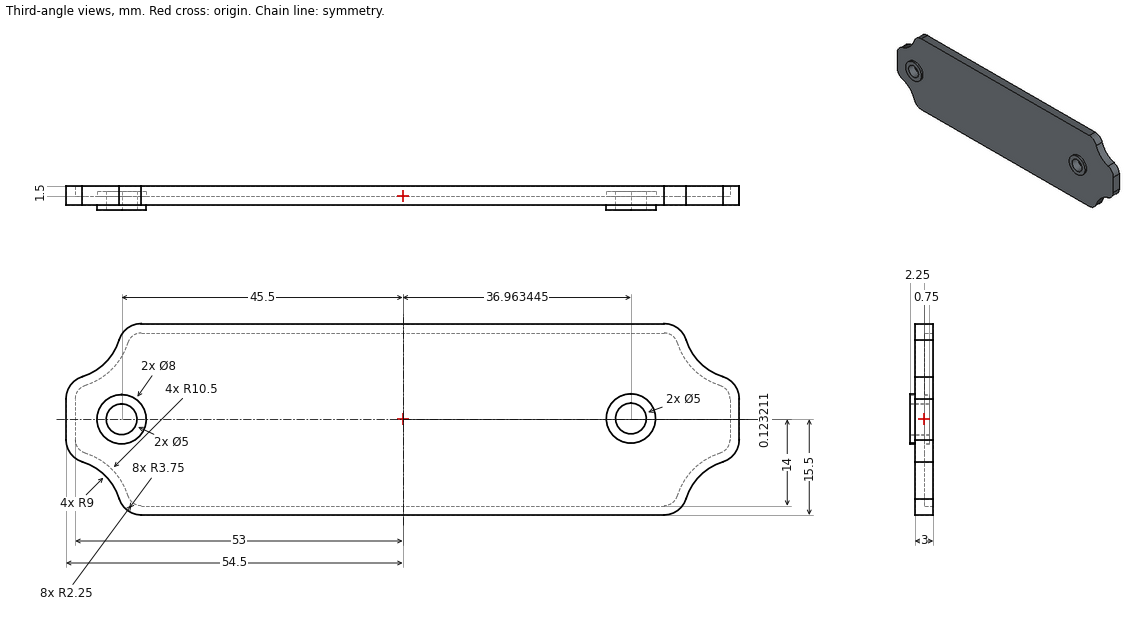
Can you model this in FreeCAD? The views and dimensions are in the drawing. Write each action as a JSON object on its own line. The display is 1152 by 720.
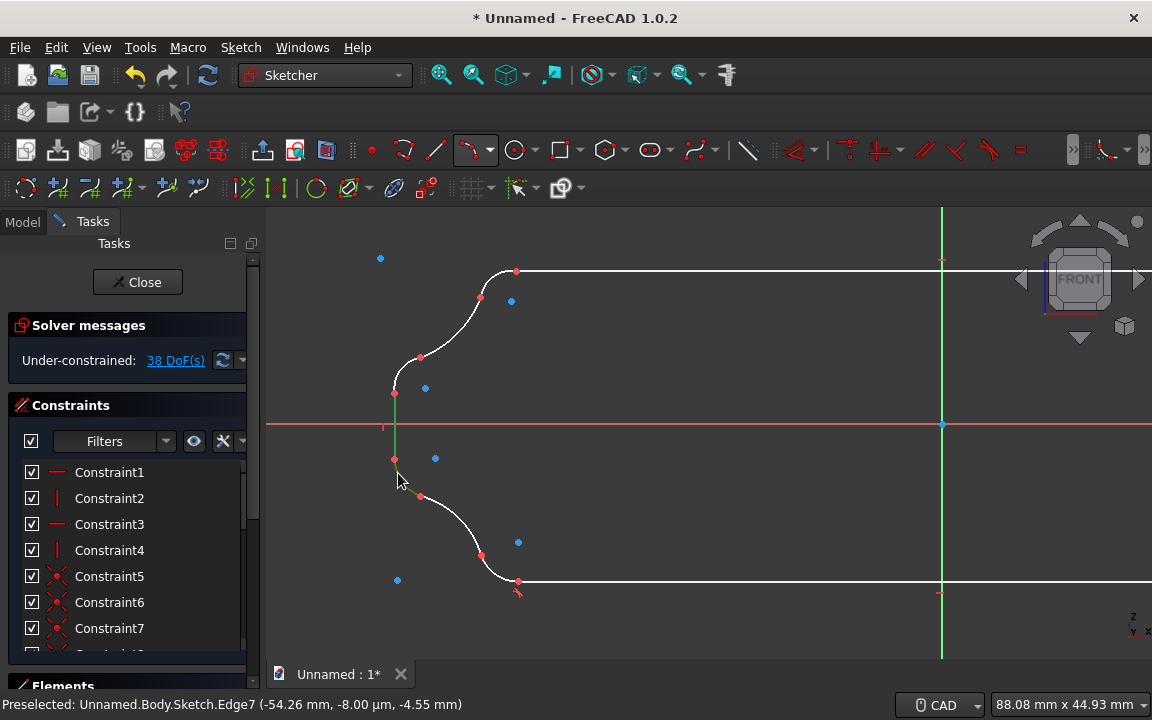
{"action": "left_click", "coordinate": [990, 150]}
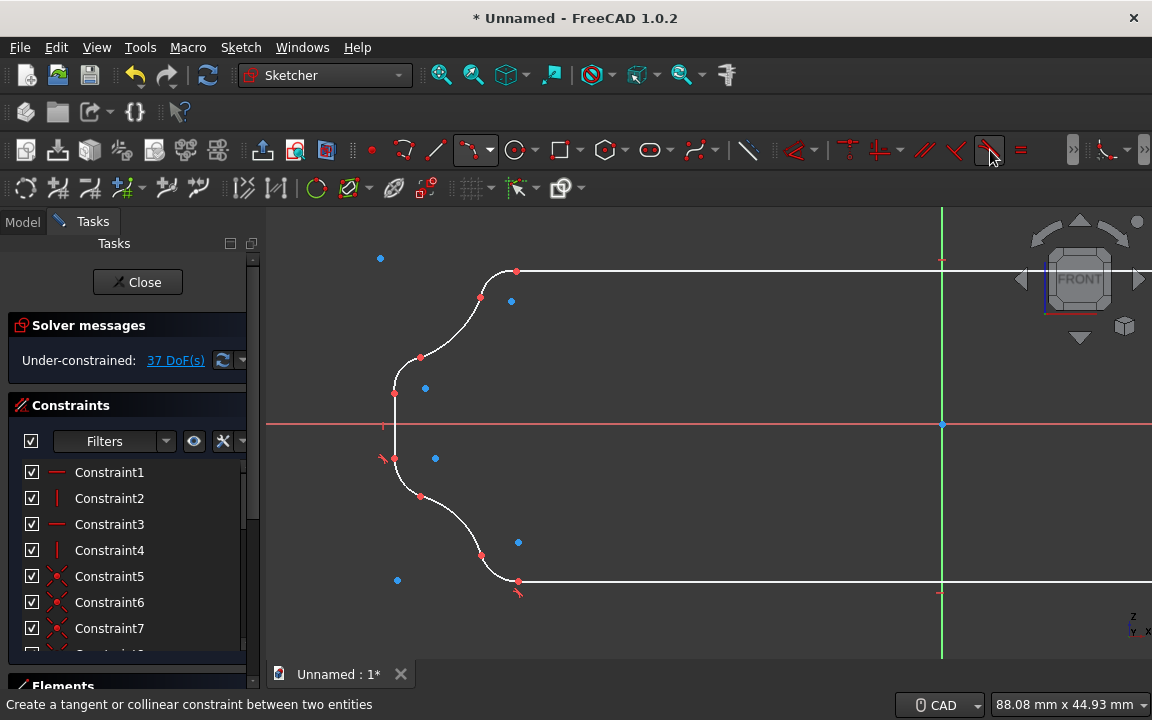
{"action": "left_click", "coordinate": [395, 439]}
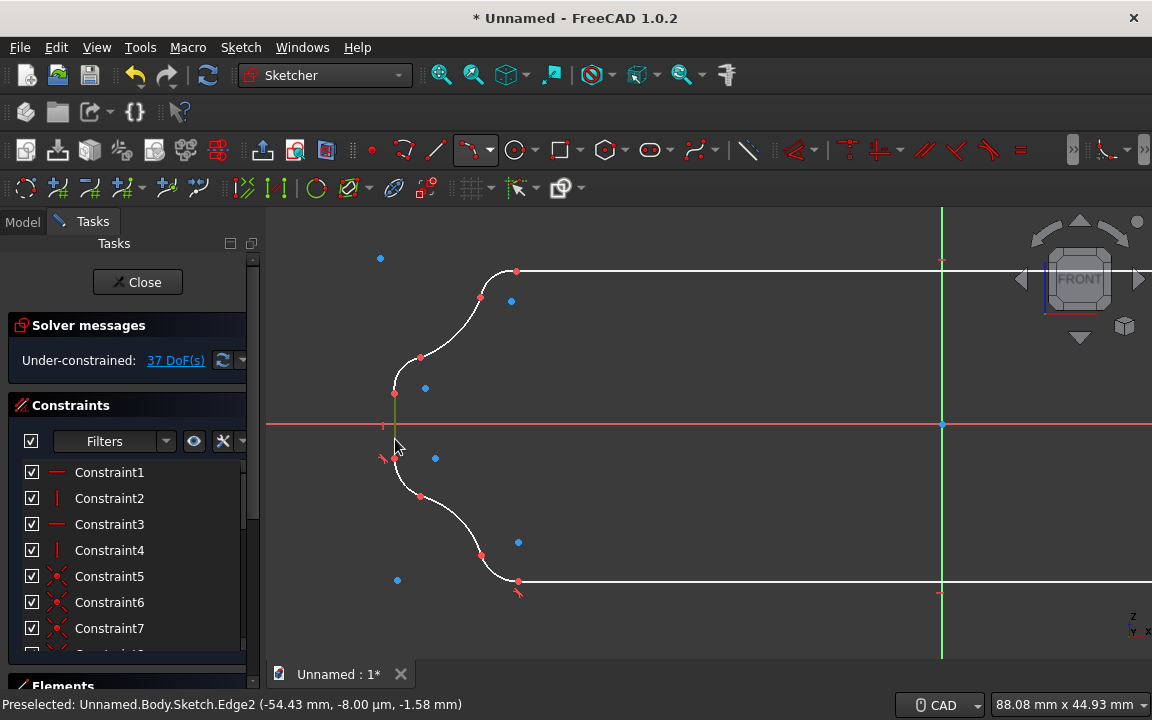
{"action": "left_click", "coordinate": [407, 363]}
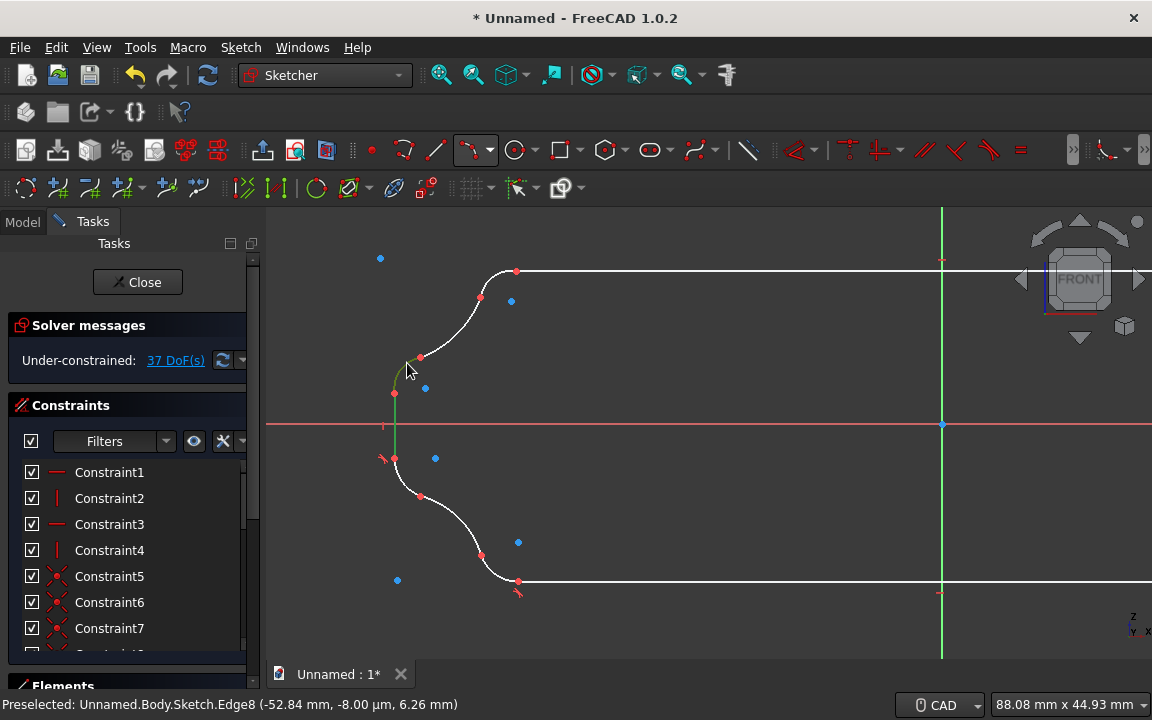
{"action": "left_click", "coordinate": [990, 150]}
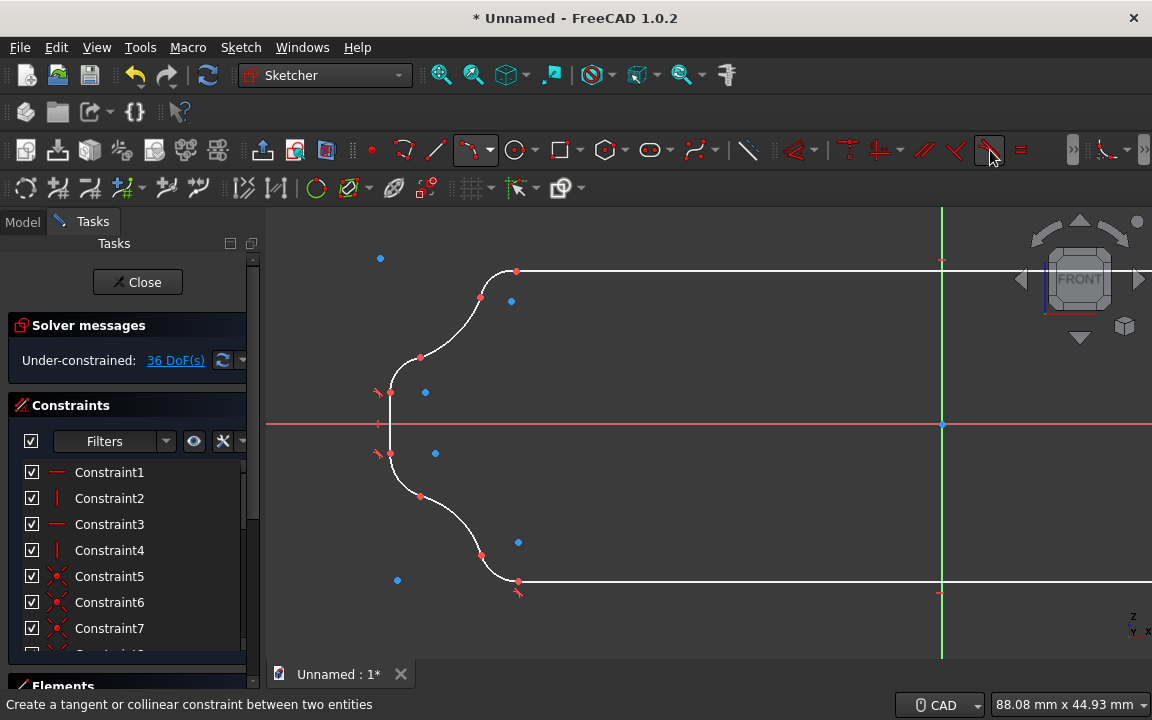
{"action": "left_click", "coordinate": [772, 271]}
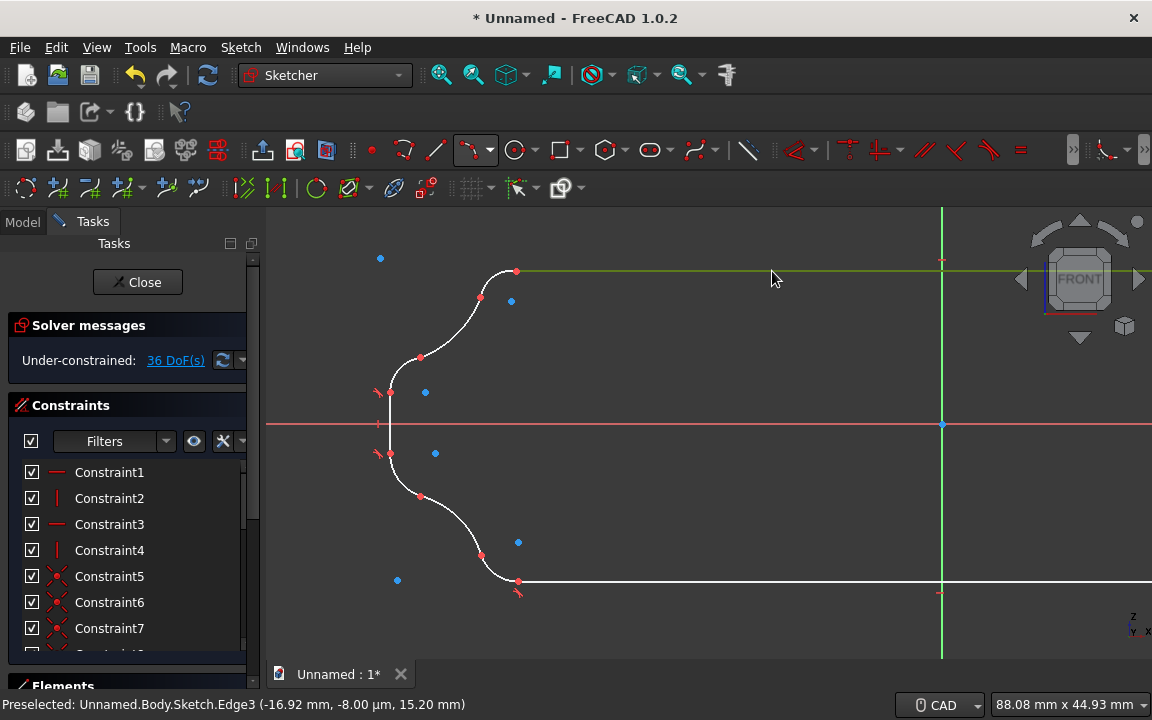
{"action": "left_click", "coordinate": [502, 272]}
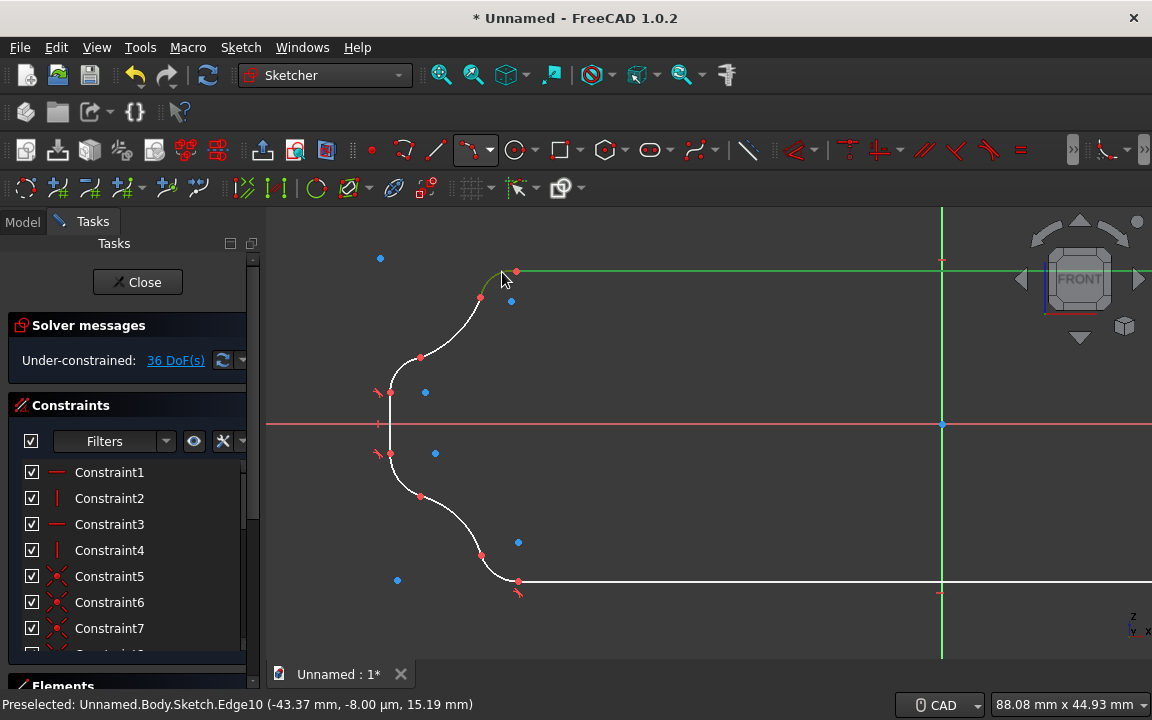
{"action": "left_click", "coordinate": [990, 150]}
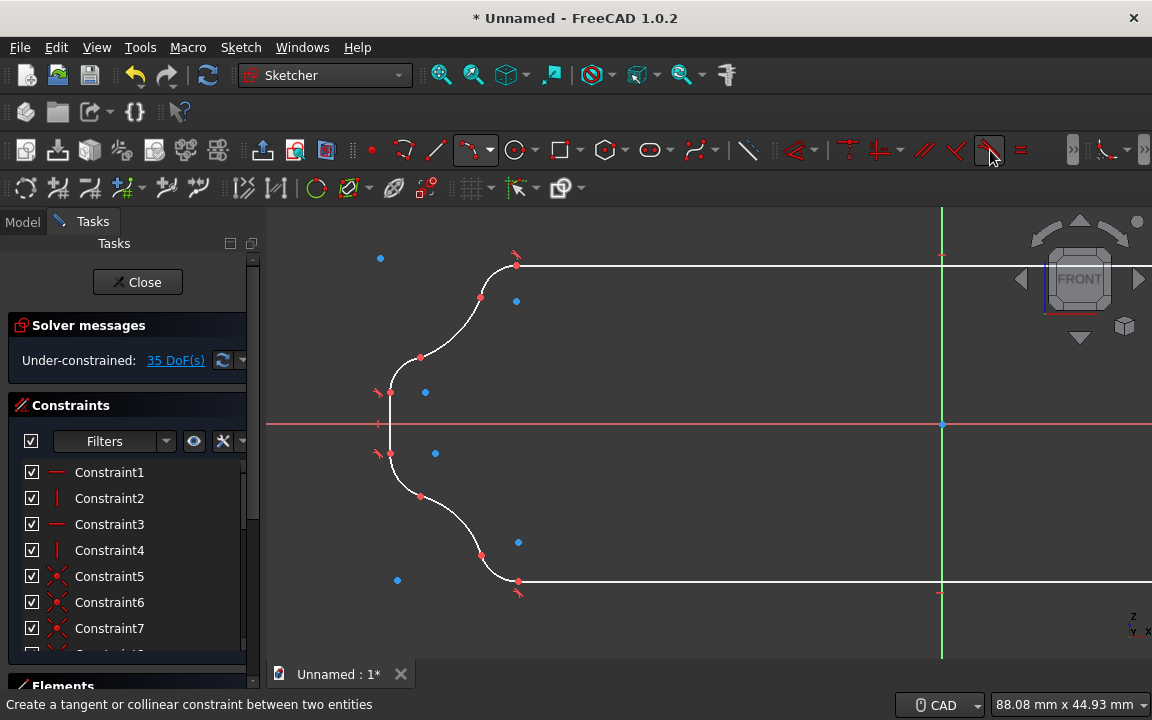
{"action": "left_click", "coordinate": [772, 266]}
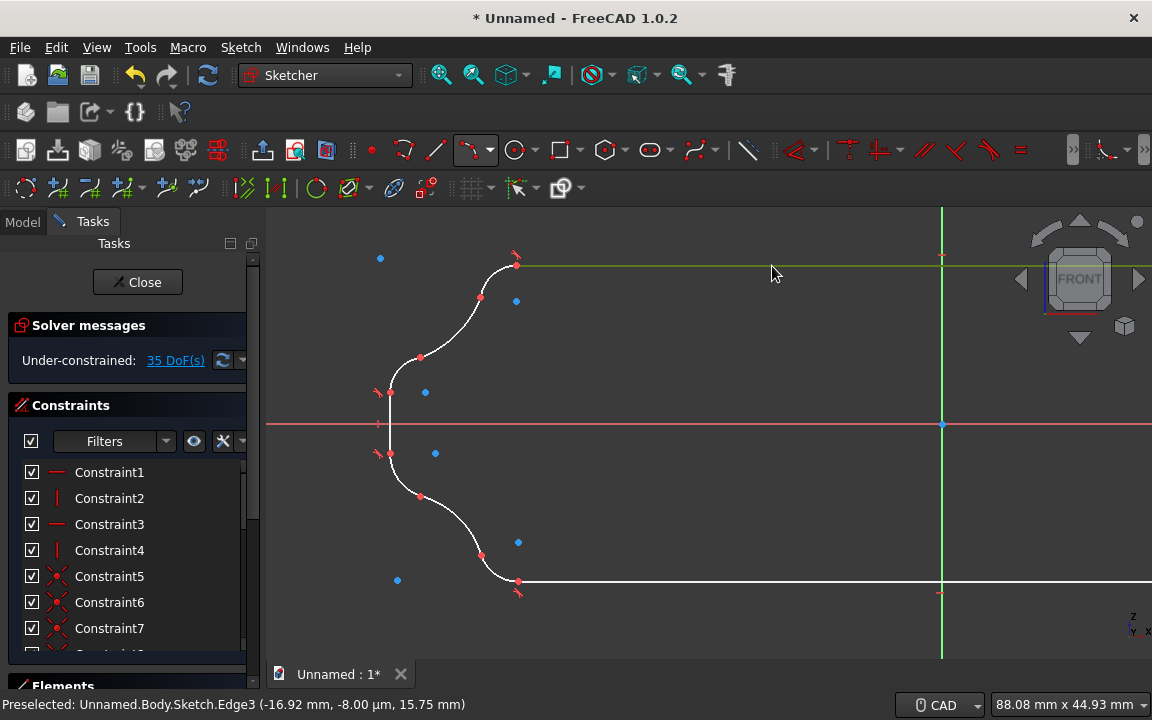
{"action": "scroll", "coordinate": [394, 440], "scroll_direction": "down", "scroll_amount": 4}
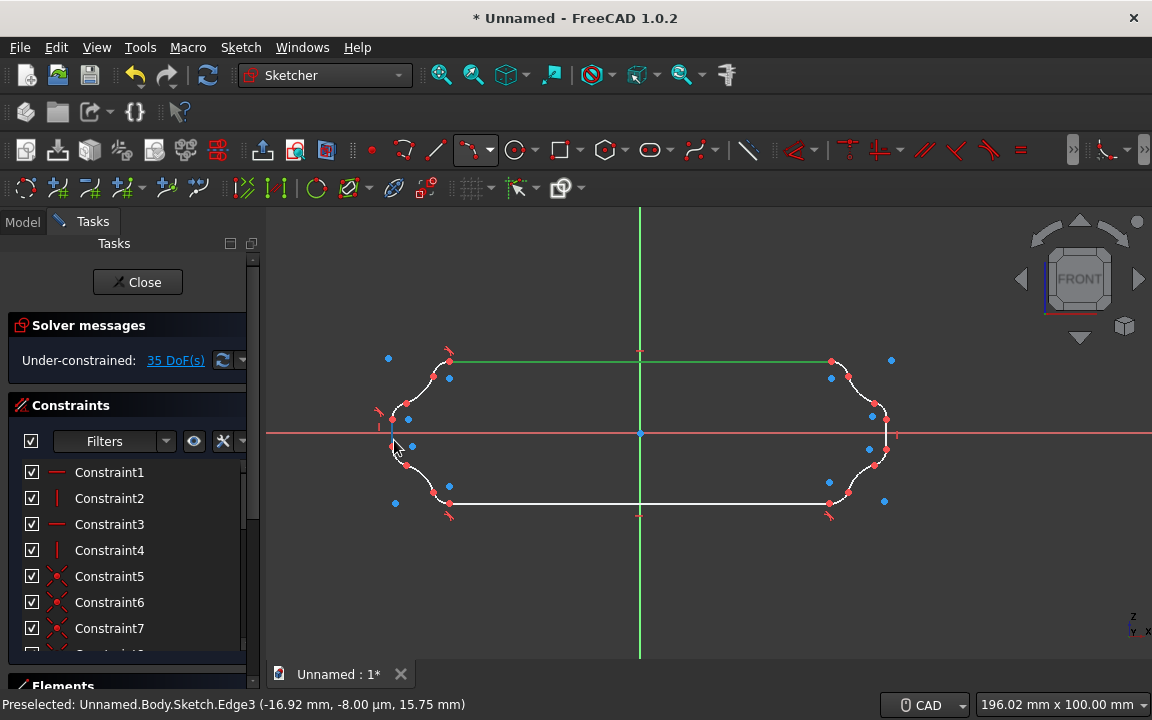
{"action": "scroll", "coordinate": [846, 370], "scroll_direction": "up", "scroll_amount": 4}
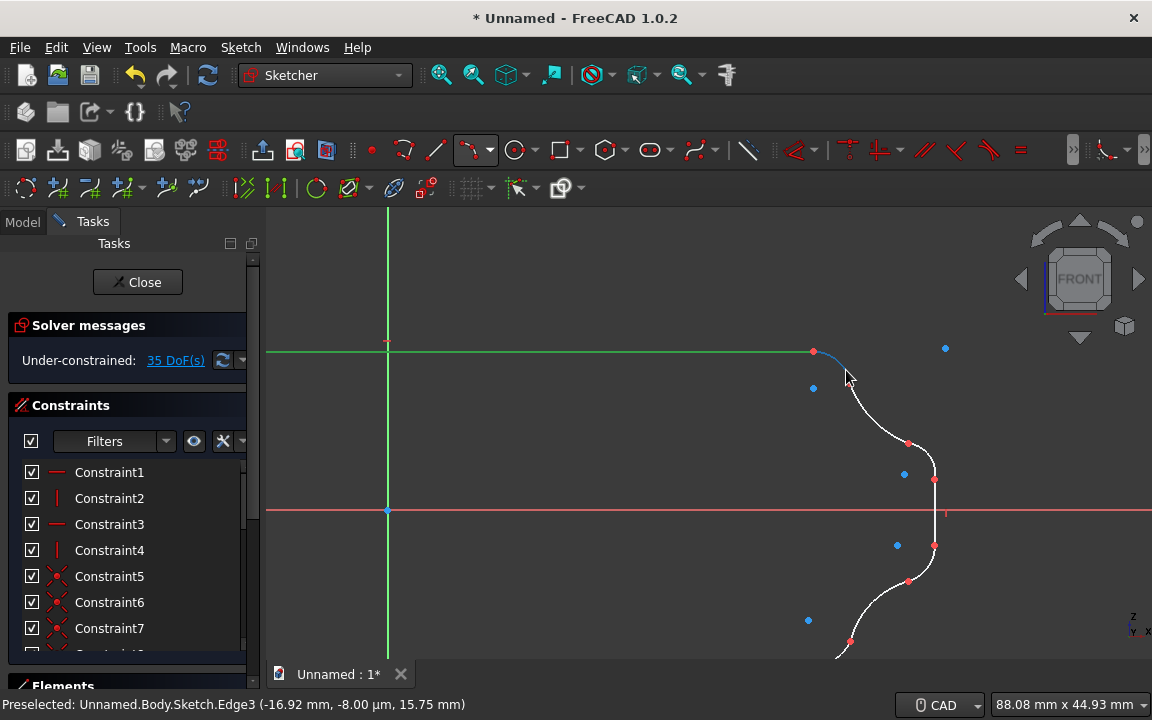
{"action": "left_click", "coordinate": [844, 369]}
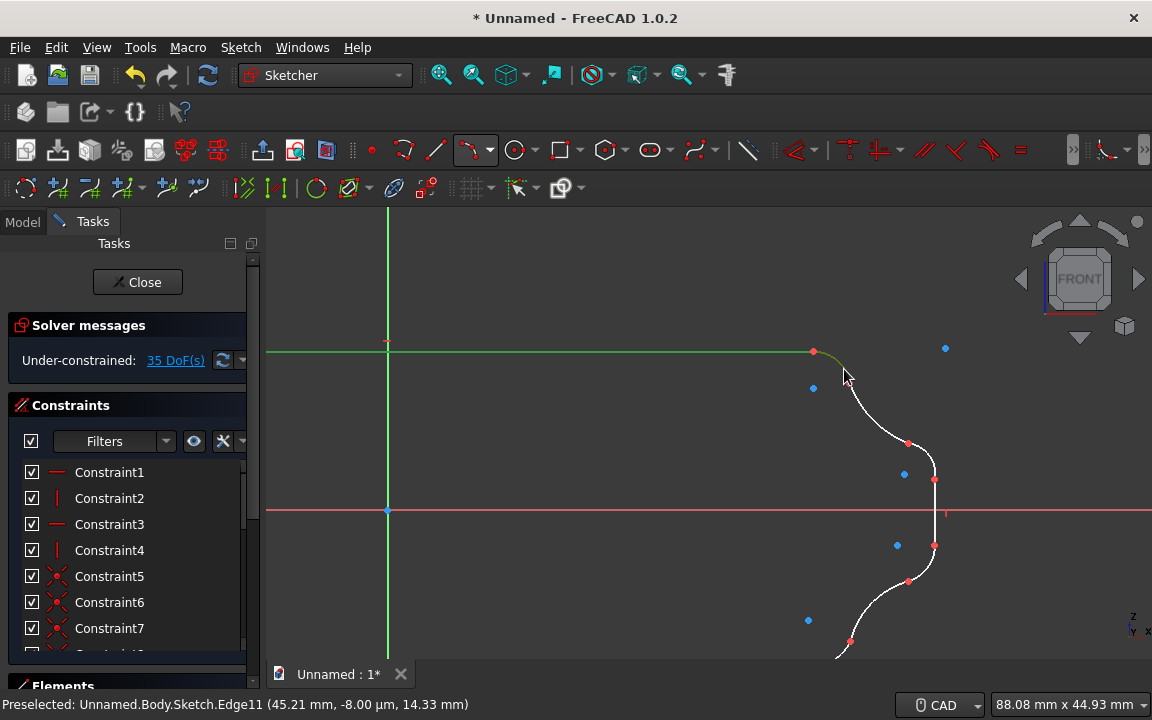
{"action": "left_click", "coordinate": [990, 150]}